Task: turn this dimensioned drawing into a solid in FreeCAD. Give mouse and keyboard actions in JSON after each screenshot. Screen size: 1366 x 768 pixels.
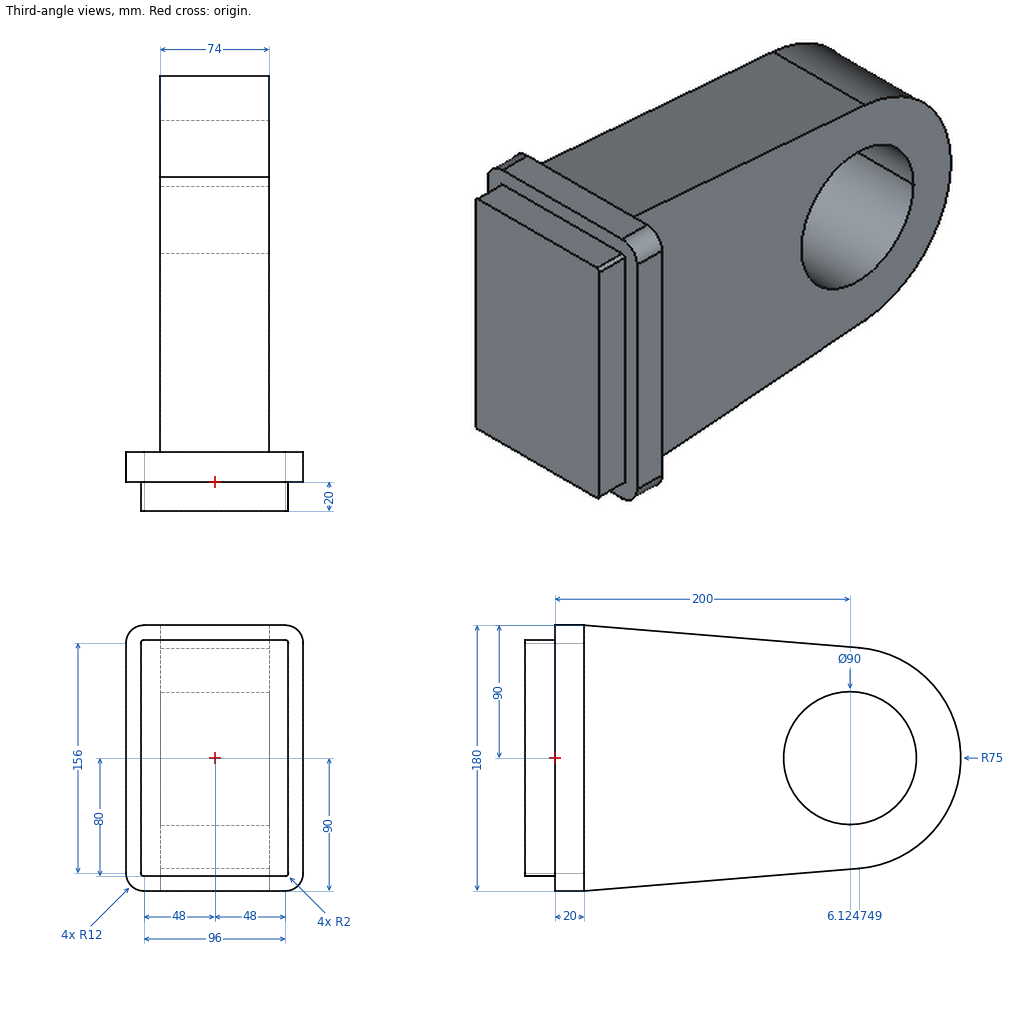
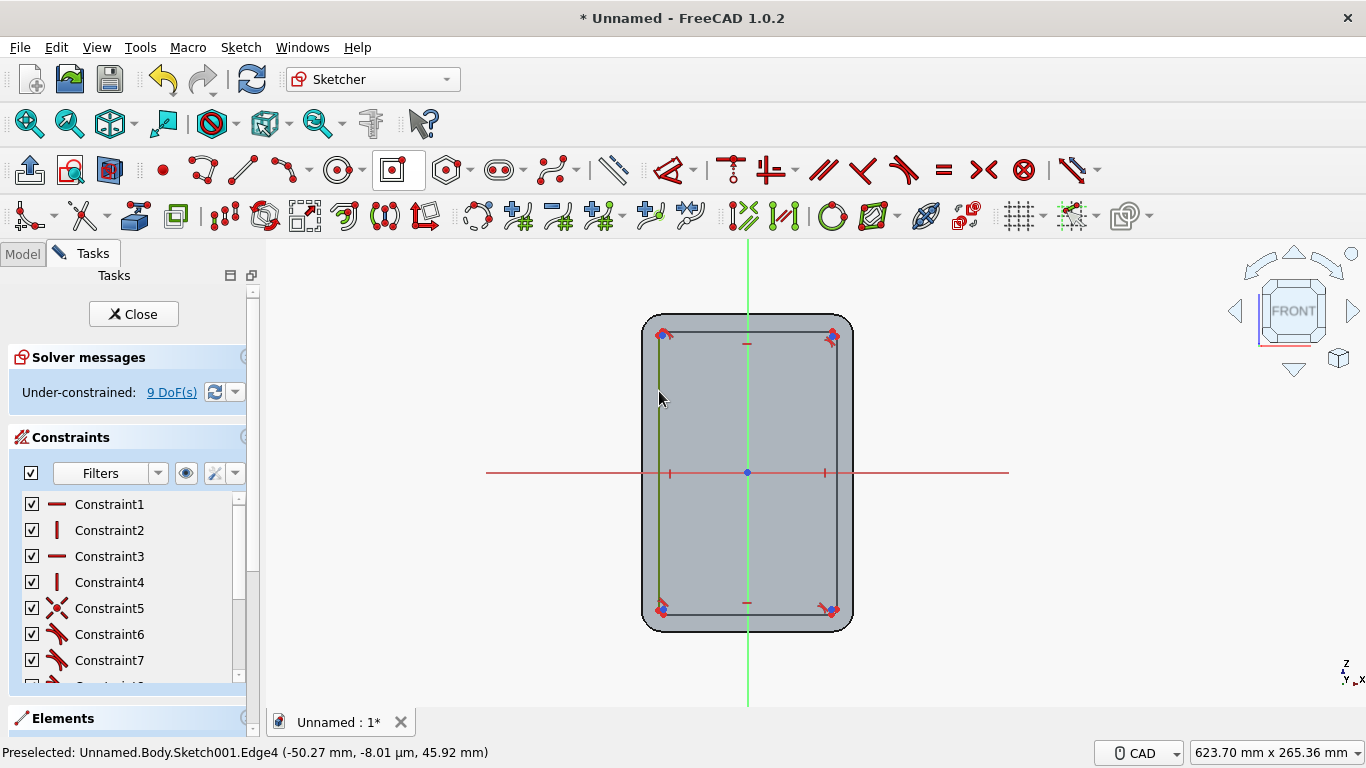
{"action": "scroll", "coordinate": [661, 614], "scroll_direction": "up", "scroll_amount": 8}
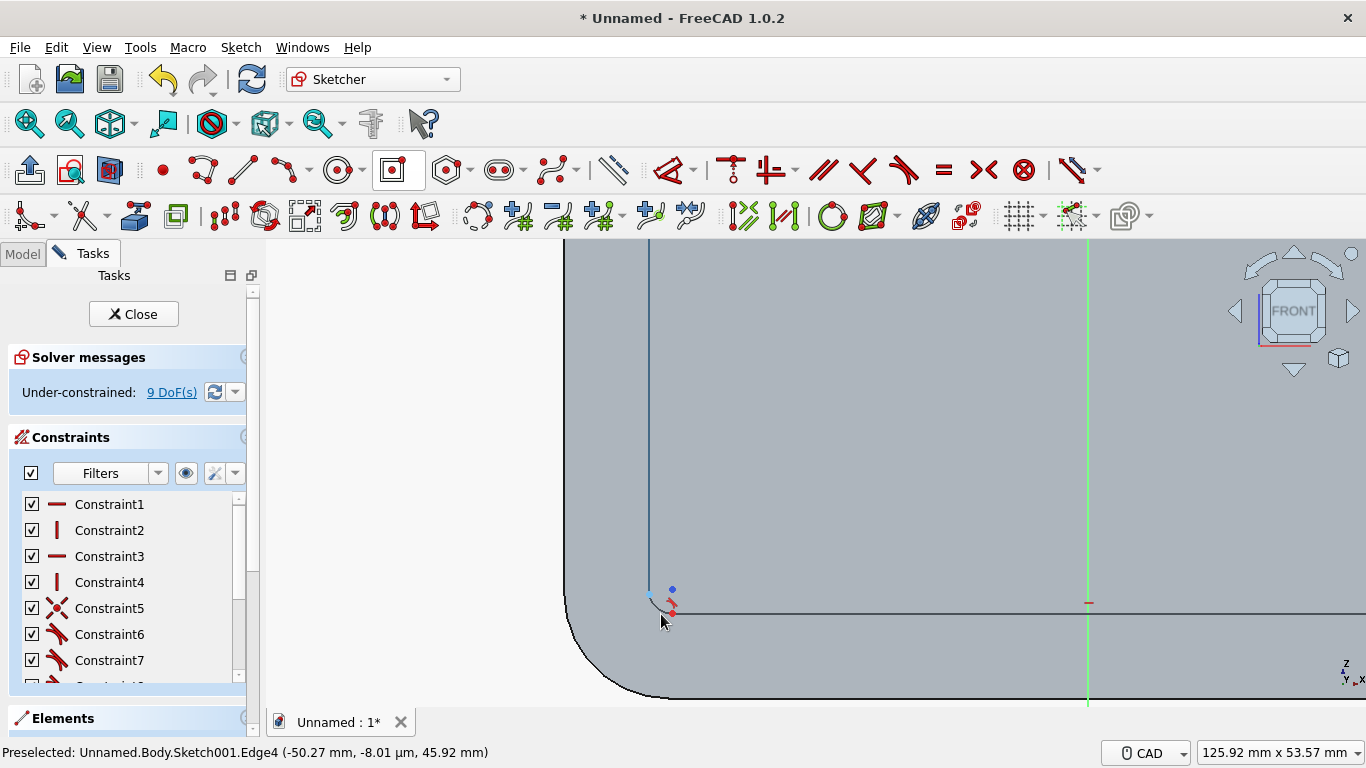
{"action": "left_click", "coordinate": [658, 608]}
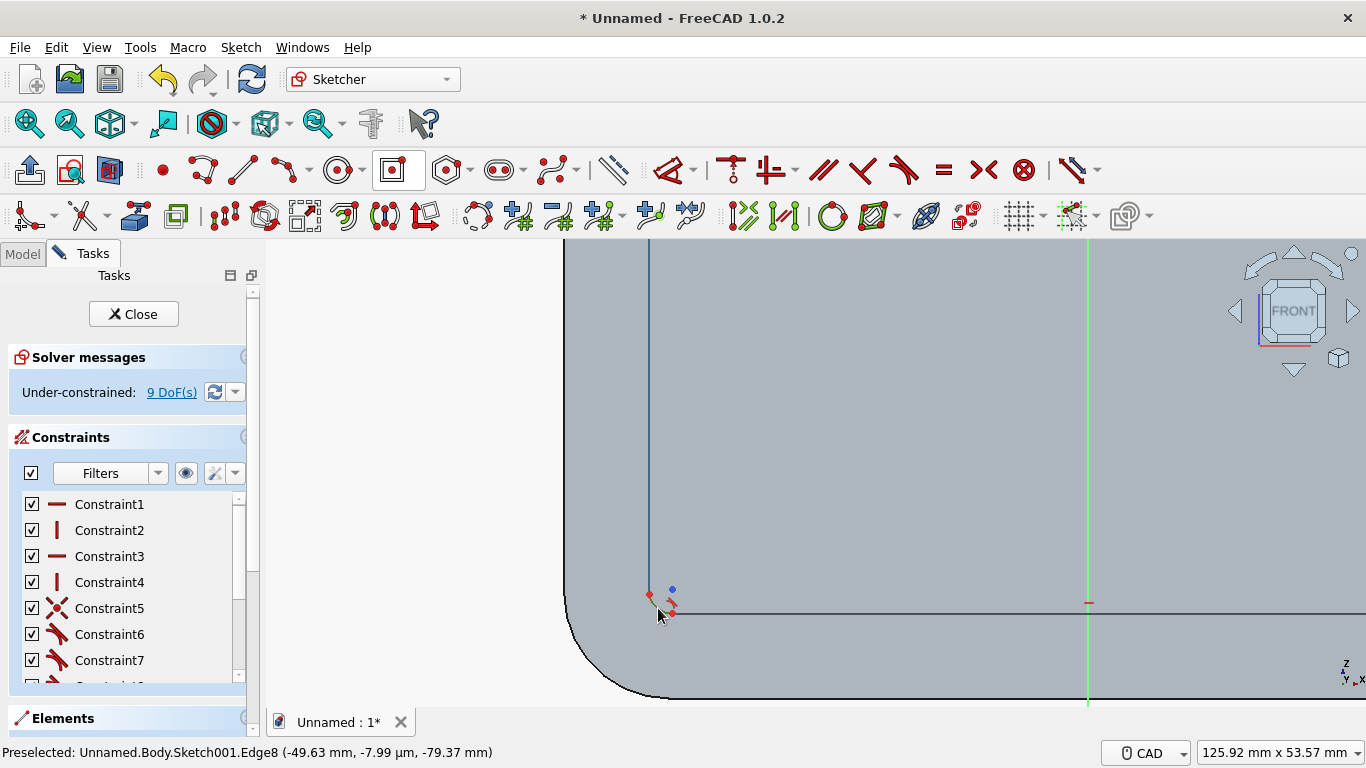
{"action": "key", "text": "t"}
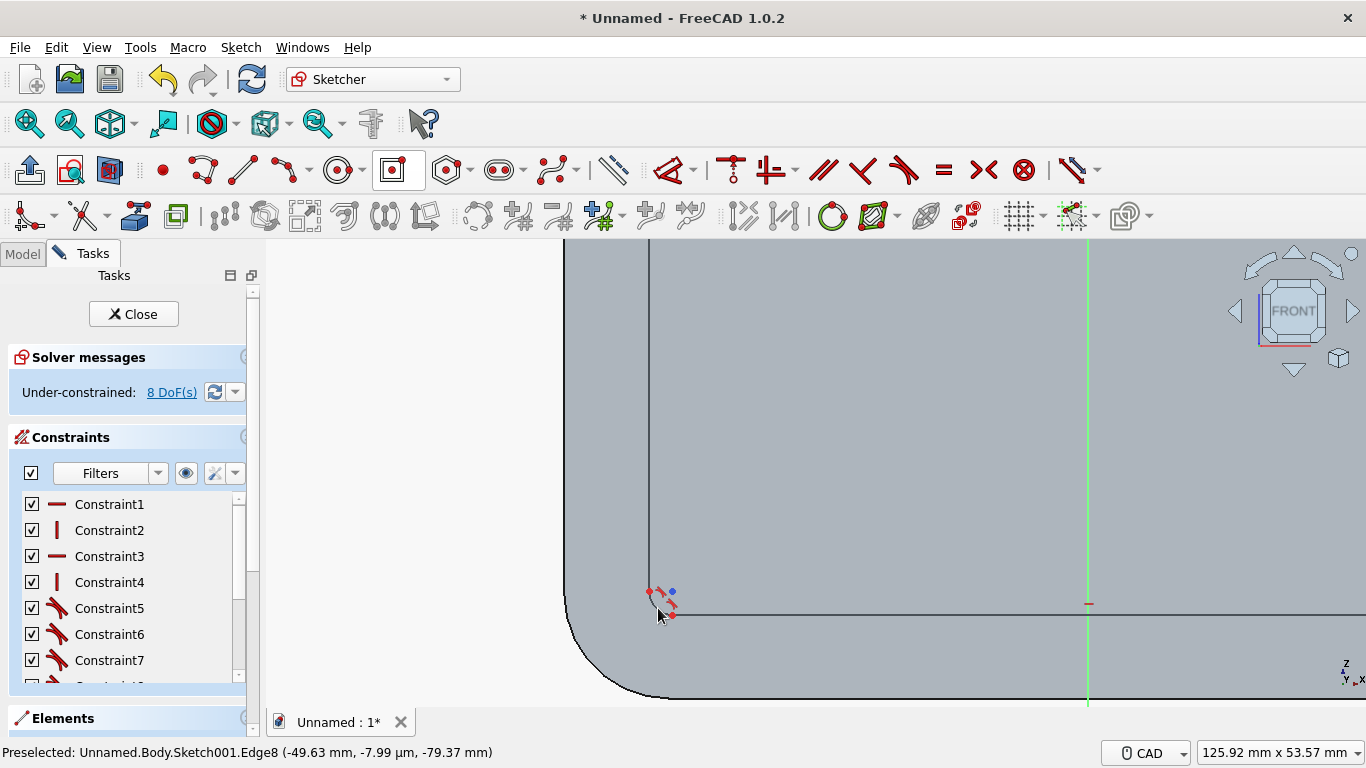
{"action": "scroll", "coordinate": [661, 615], "scroll_direction": "down", "scroll_amount": 8}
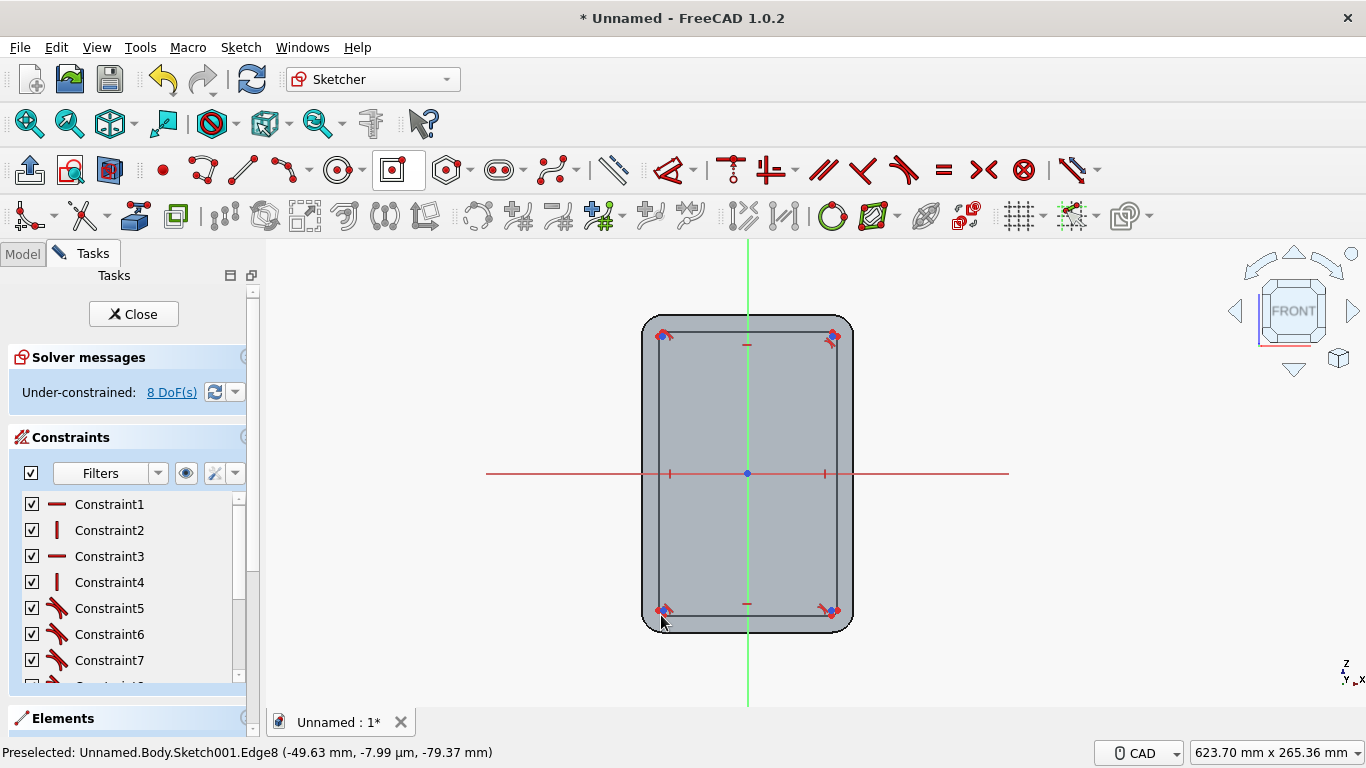
{"action": "scroll", "coordinate": [834, 615], "scroll_direction": "up", "scroll_amount": 9}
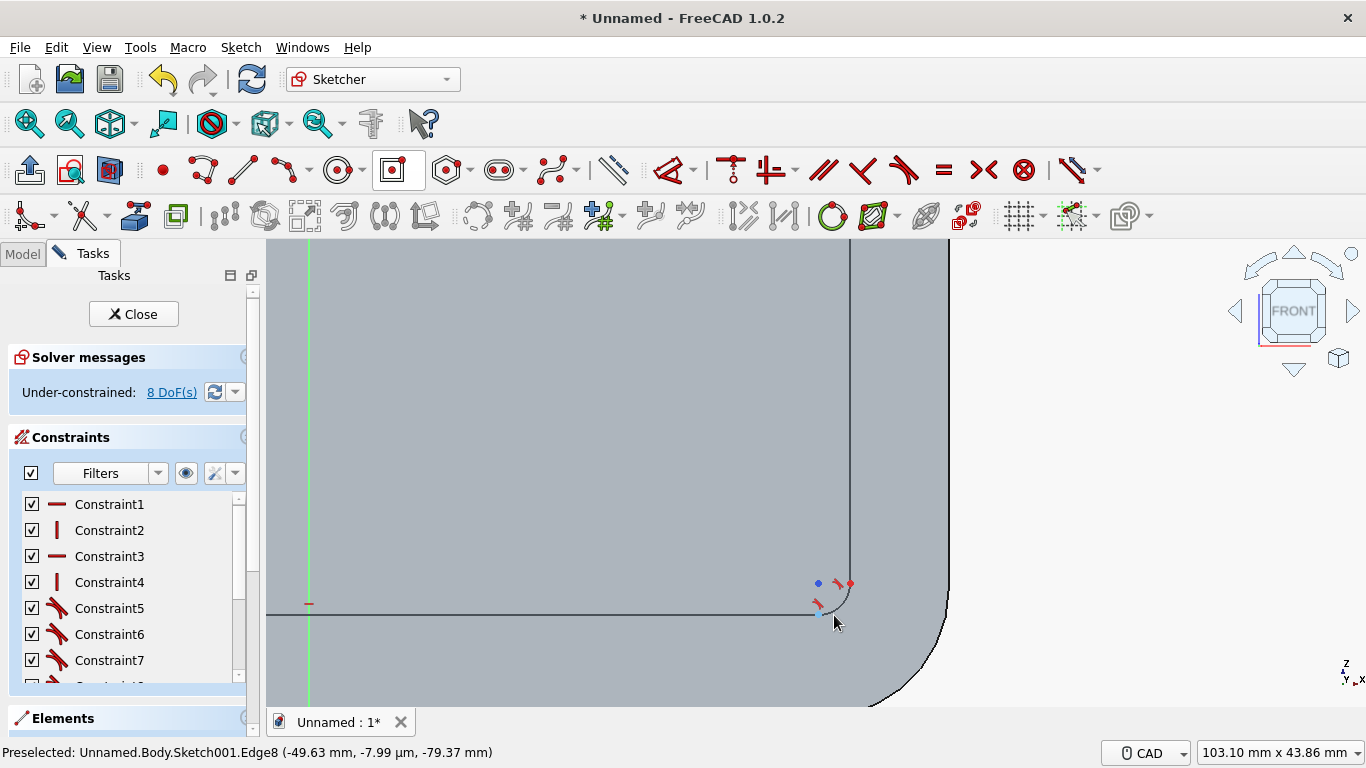
{"action": "left_click", "coordinate": [833, 612]}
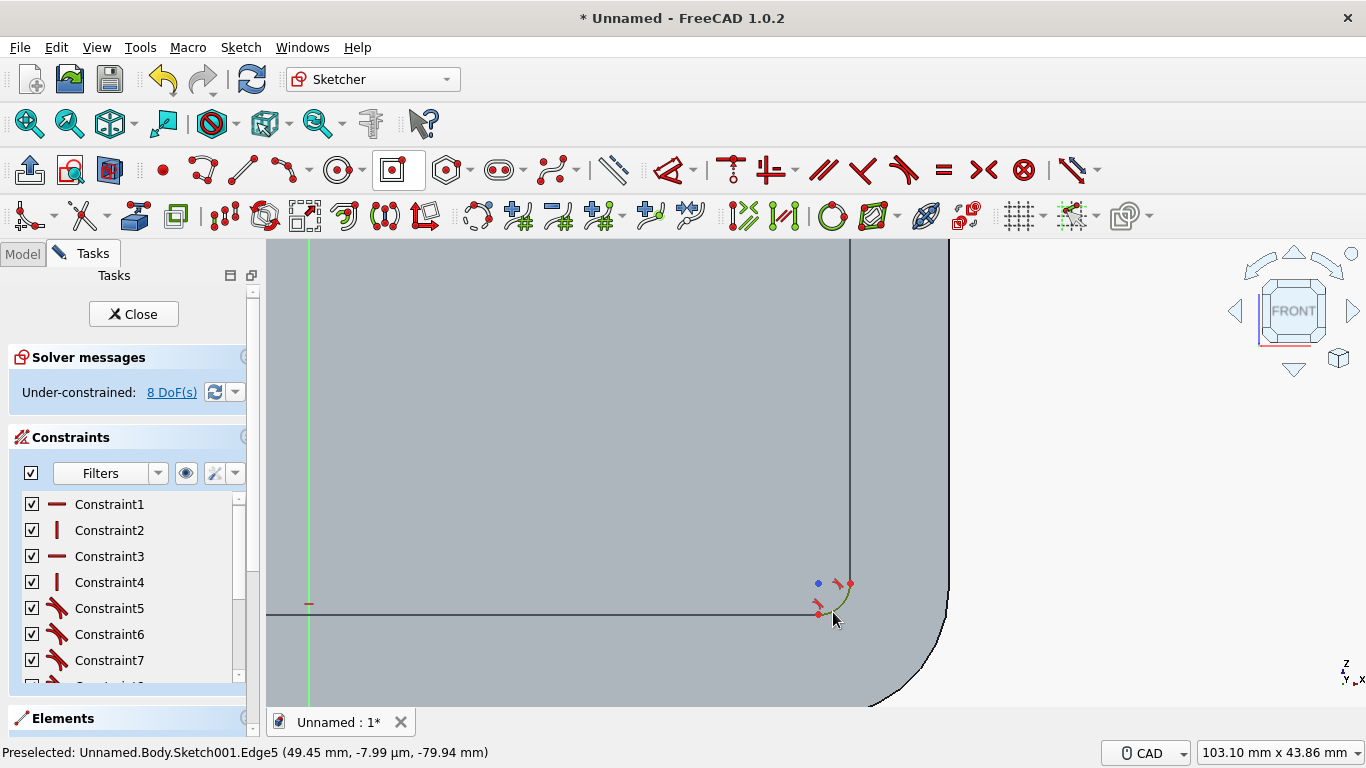
{"action": "scroll", "coordinate": [834, 615], "scroll_direction": "down", "scroll_amount": 9}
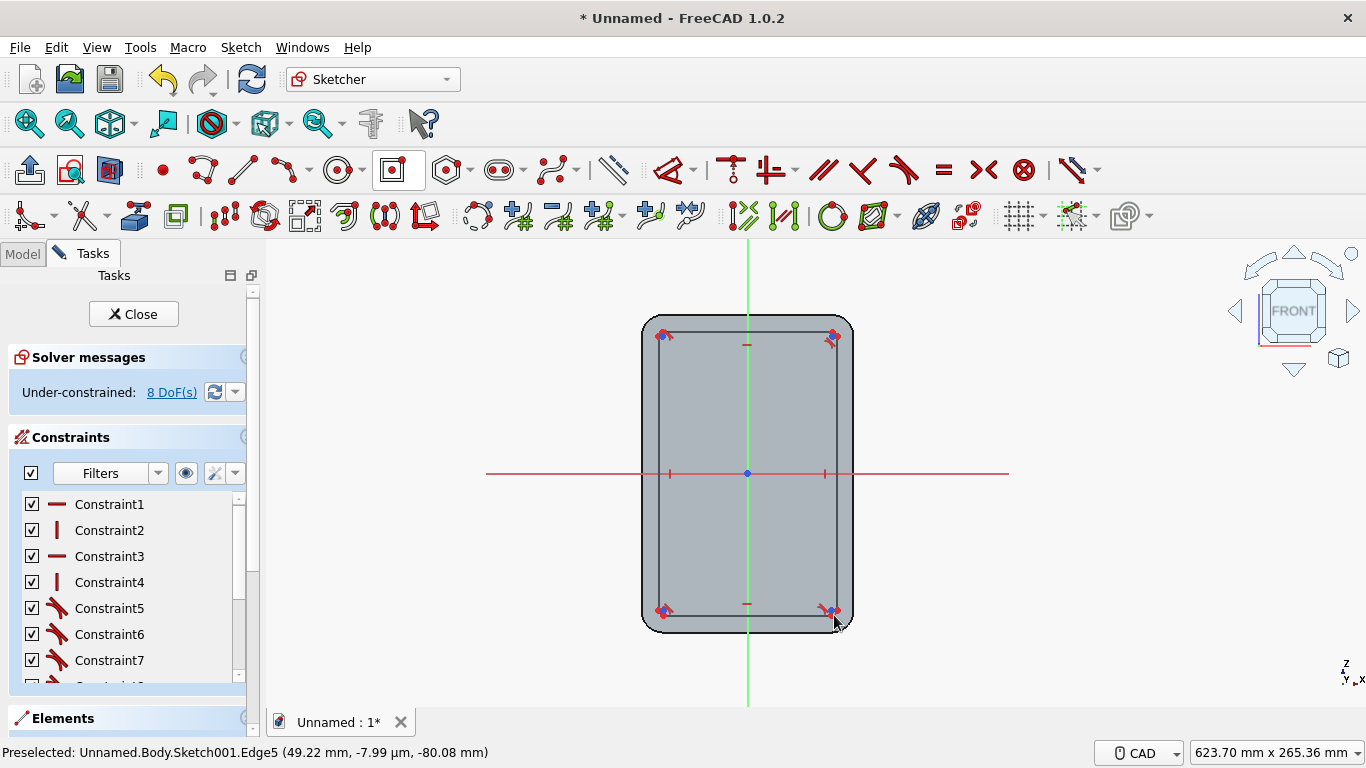
{"action": "scroll", "coordinate": [837, 335], "scroll_direction": "up", "scroll_amount": 10}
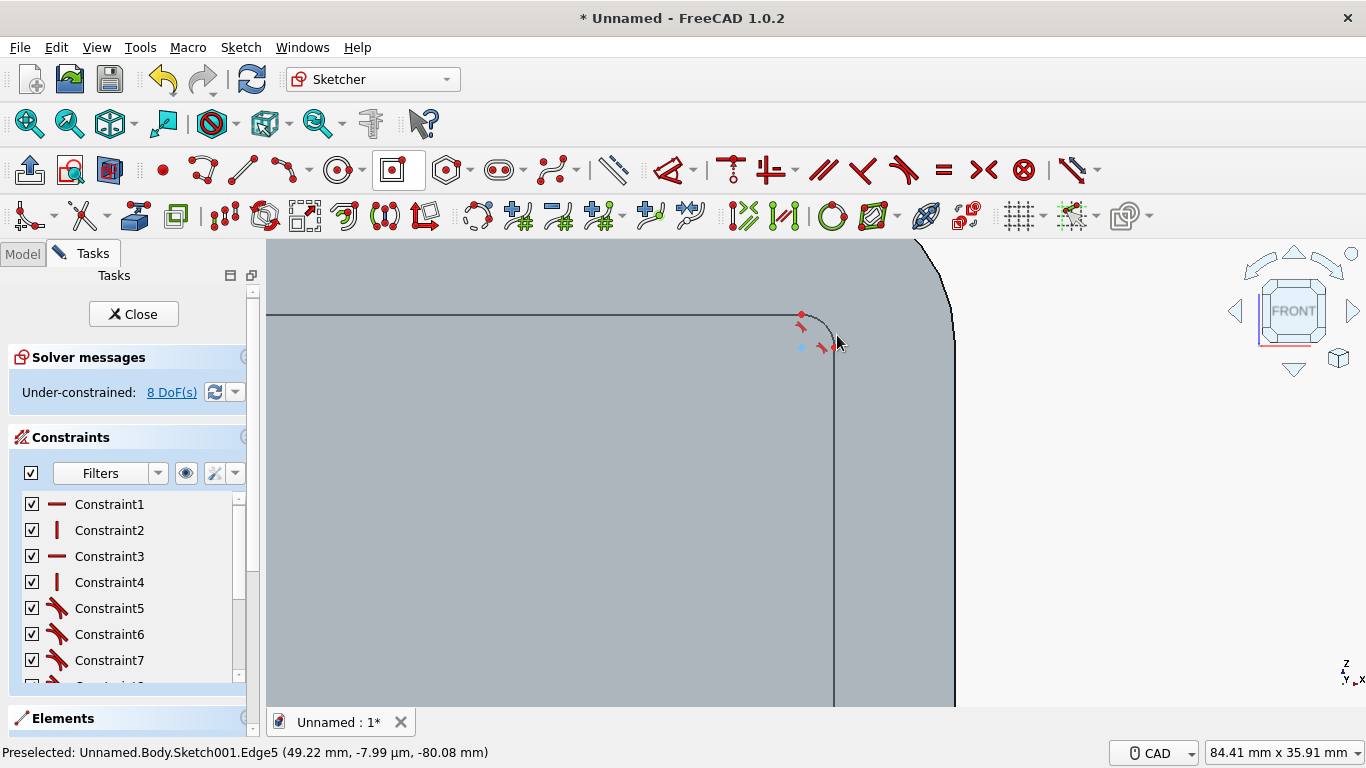
{"action": "left_click", "coordinate": [831, 333]}